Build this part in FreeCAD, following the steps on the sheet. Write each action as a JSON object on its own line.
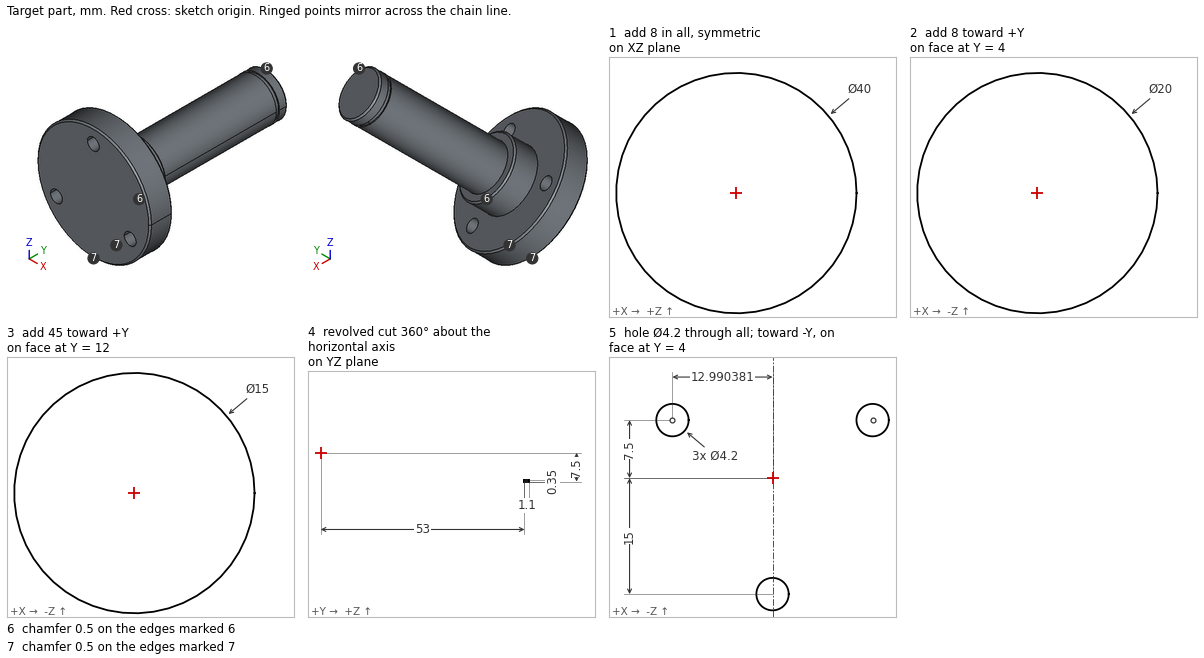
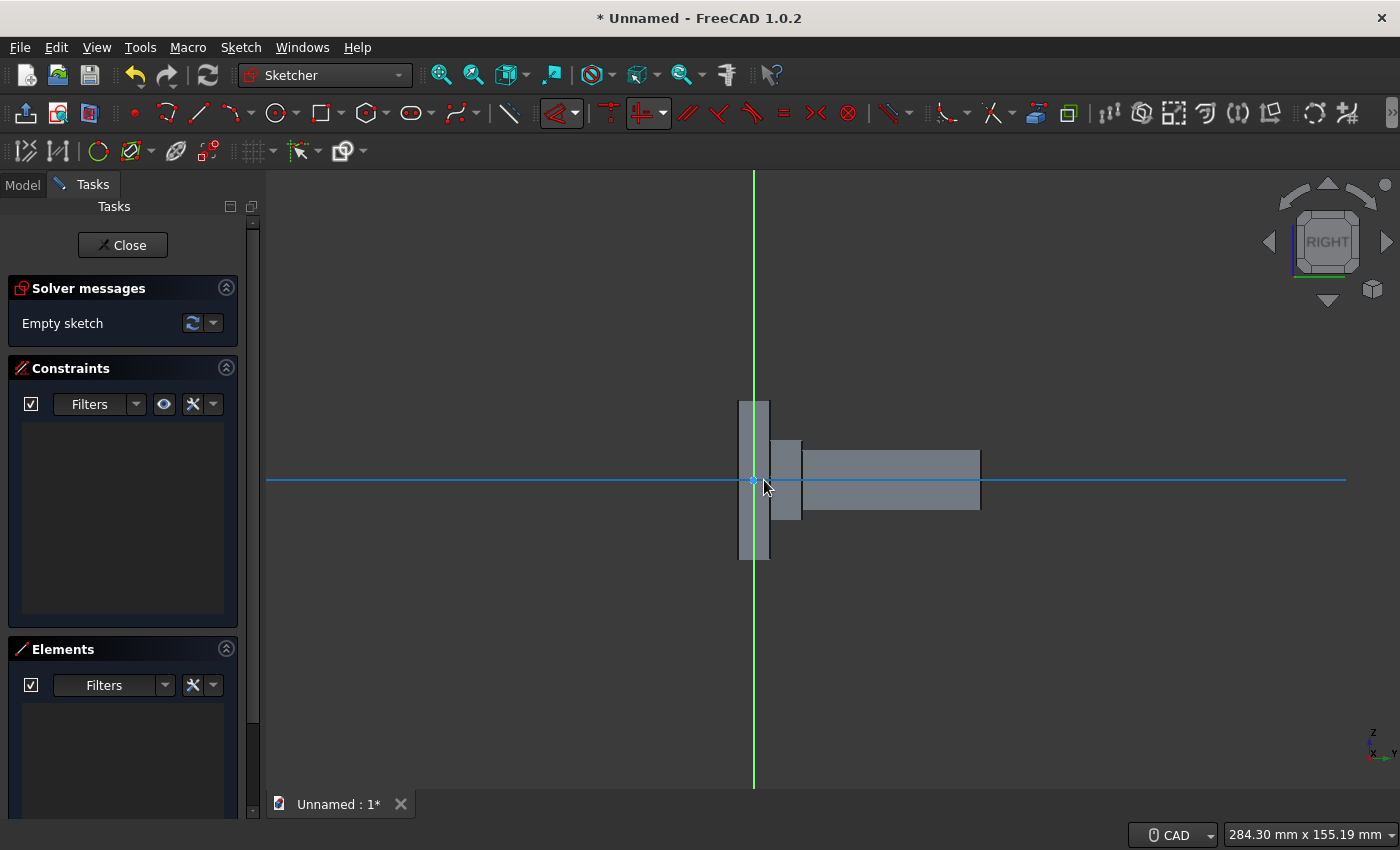
{"action": "scroll", "coordinate": [978, 511], "scroll_direction": "up", "scroll_amount": 15}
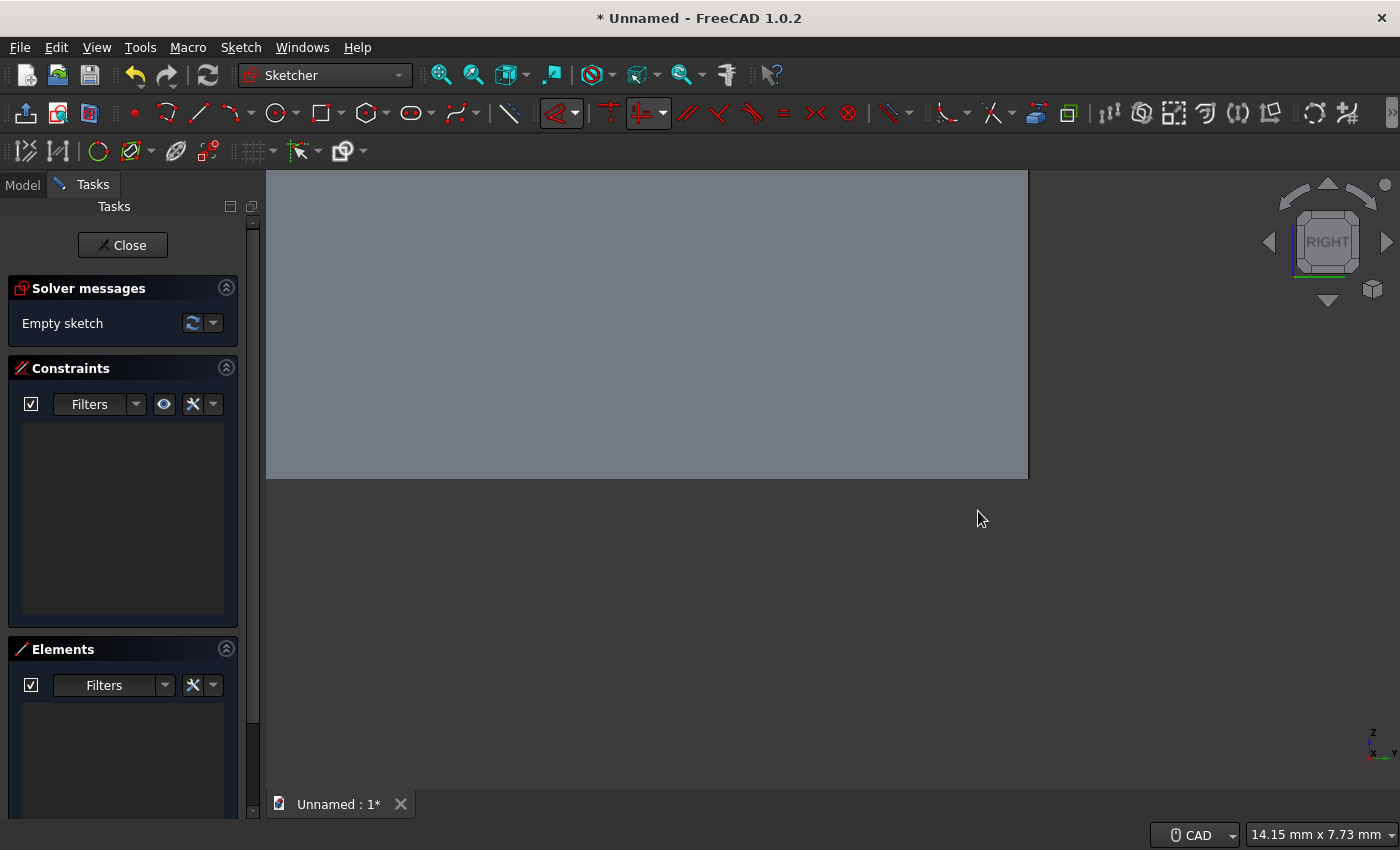
{"action": "scroll", "coordinate": [750, 465], "scroll_direction": "up", "scroll_amount": 10}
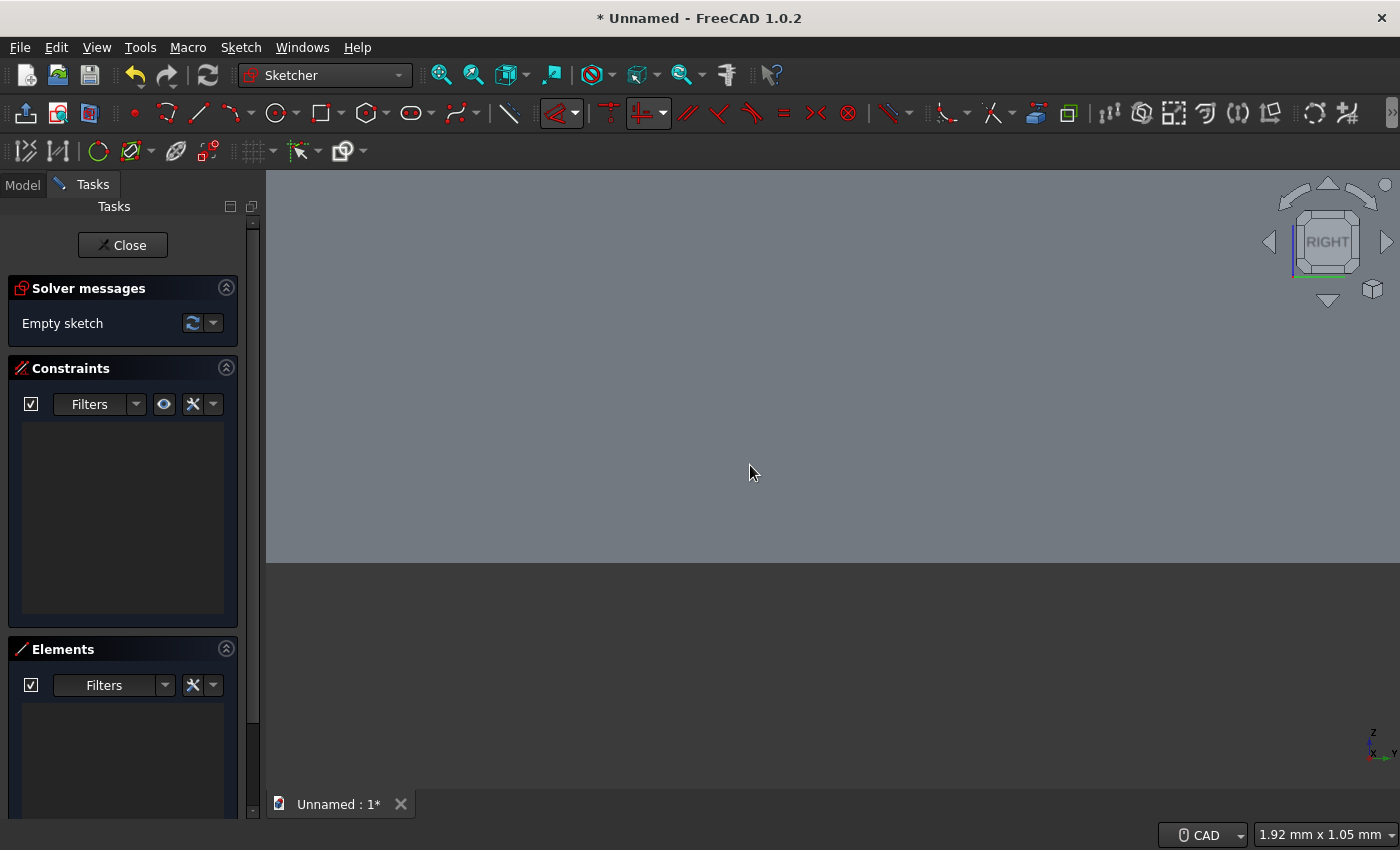
{"action": "left_click", "coordinate": [322, 114]}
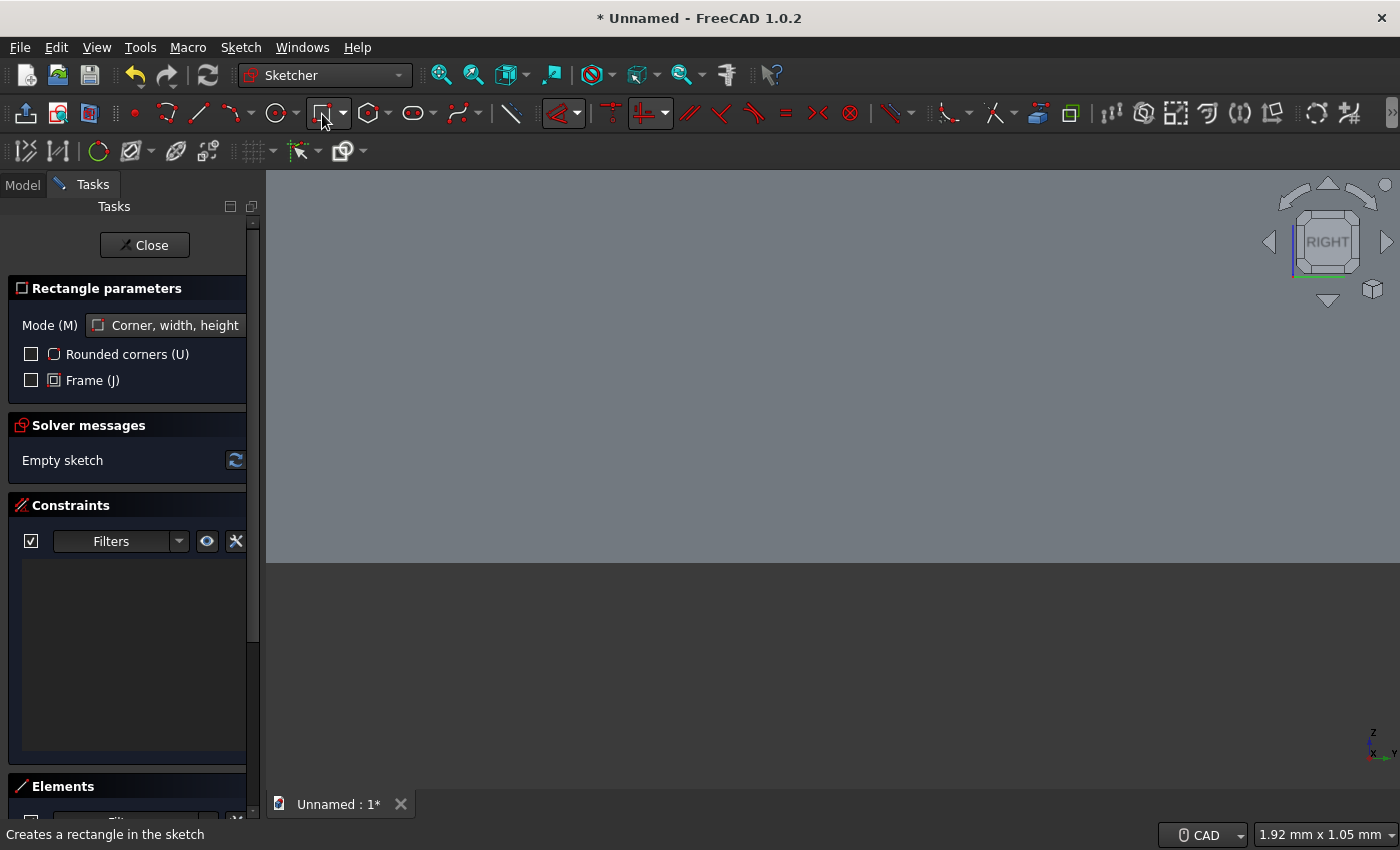
{"action": "left_click", "coordinate": [438, 376]}
{"action": "mouse_move", "coordinate": [1090, 583]}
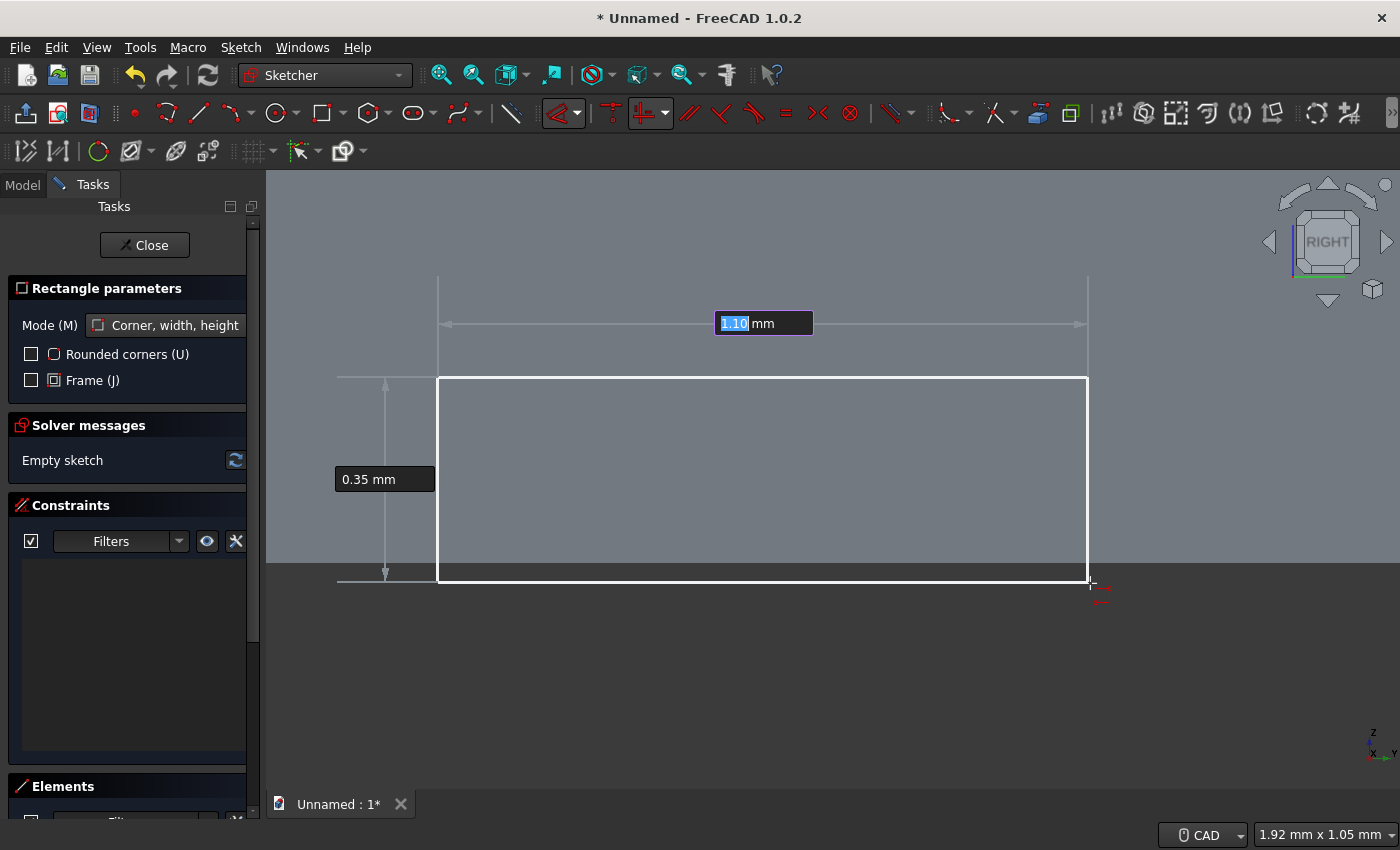
{"action": "type", "text": "1.1"}
{"action": "key", "text": "Tab"}
{"action": "type", "text": "0.35"}
{"action": "key", "text": "Return"}
{"action": "key", "text": "Escape"}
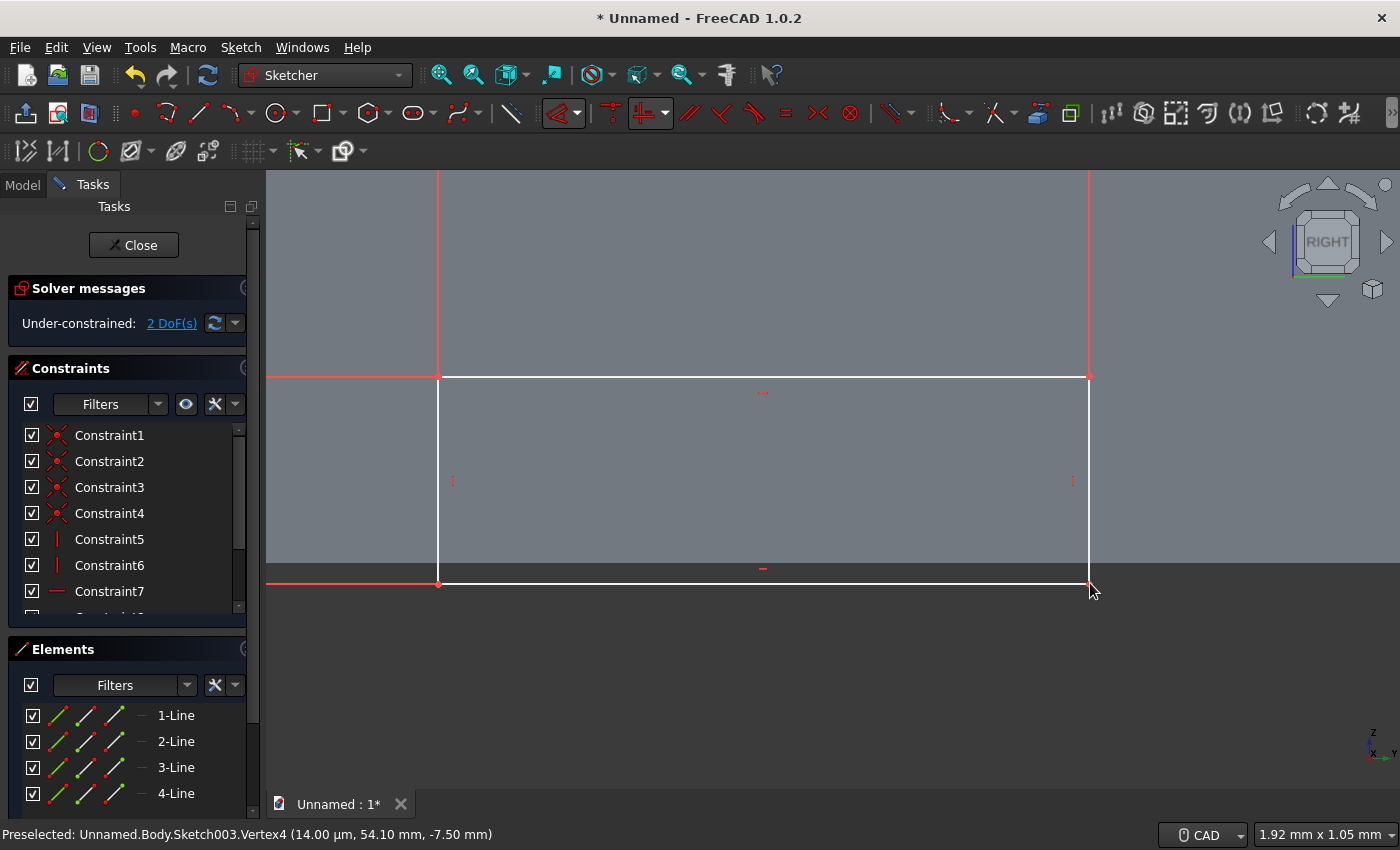
{"action": "left_click", "coordinate": [558, 114]}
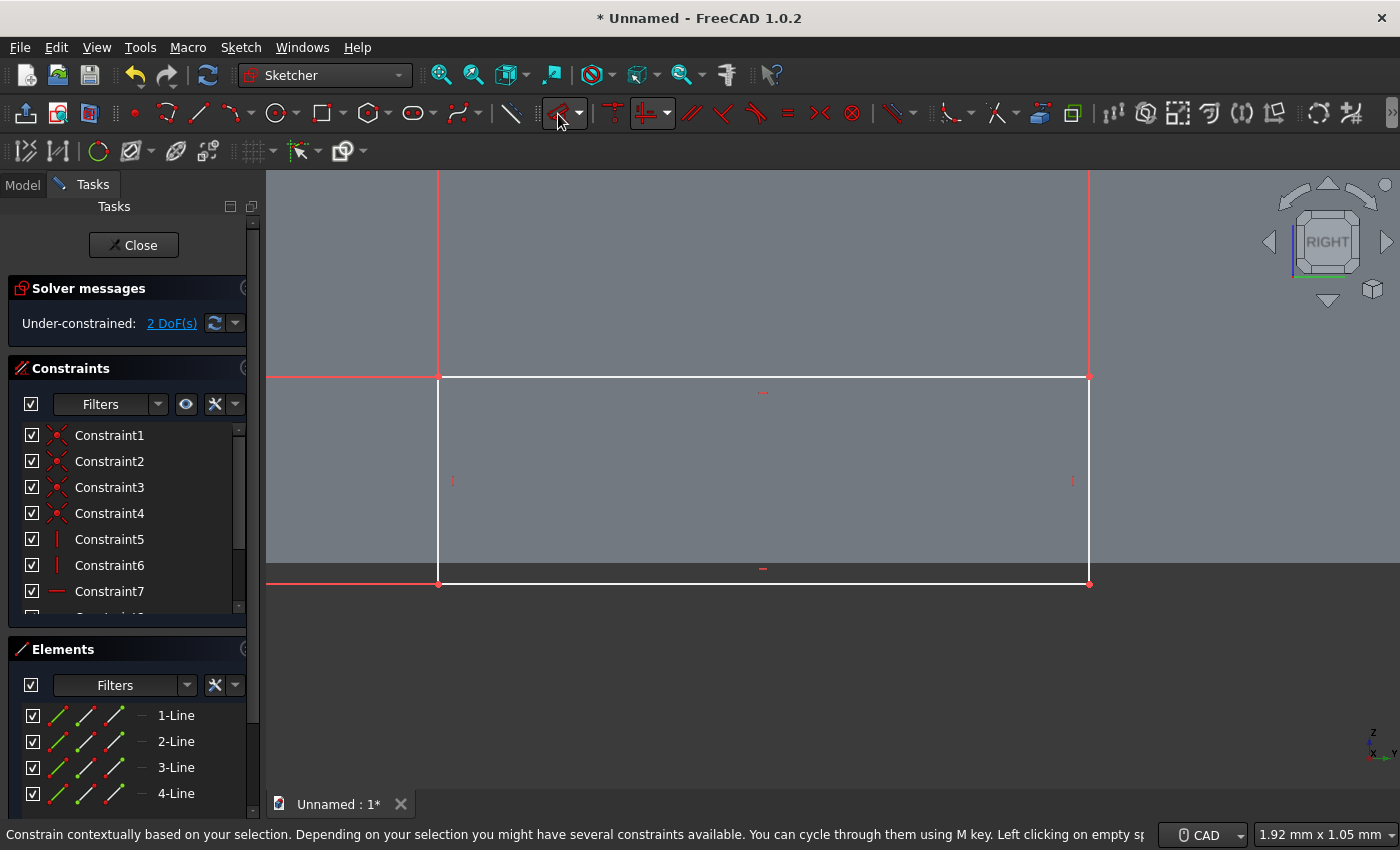
{"action": "left_click", "coordinate": [438, 377]}
{"action": "left_click", "coordinate": [366, 411]}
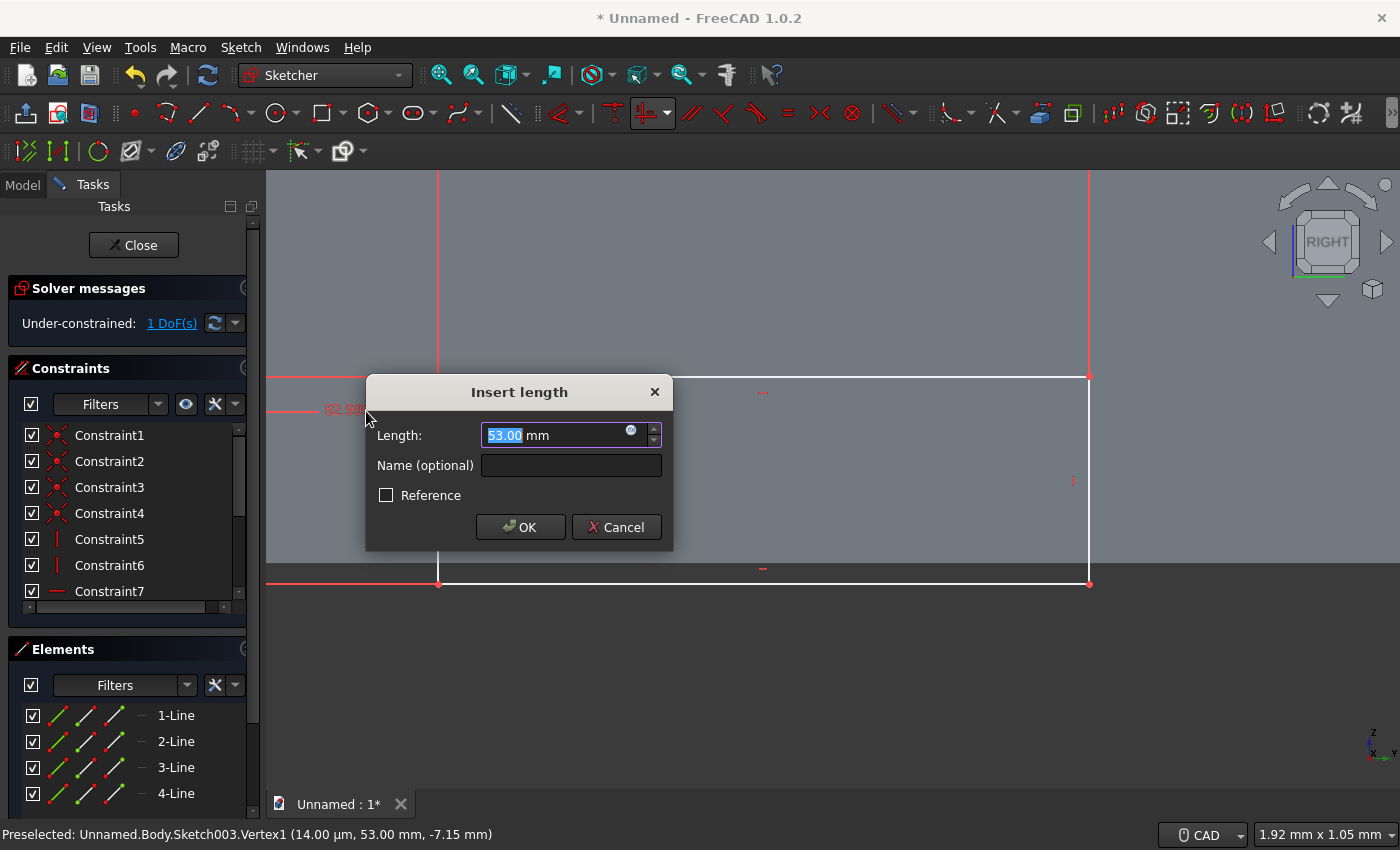
{"action": "type", "text": "53"}
{"action": "key", "text": "Return"}